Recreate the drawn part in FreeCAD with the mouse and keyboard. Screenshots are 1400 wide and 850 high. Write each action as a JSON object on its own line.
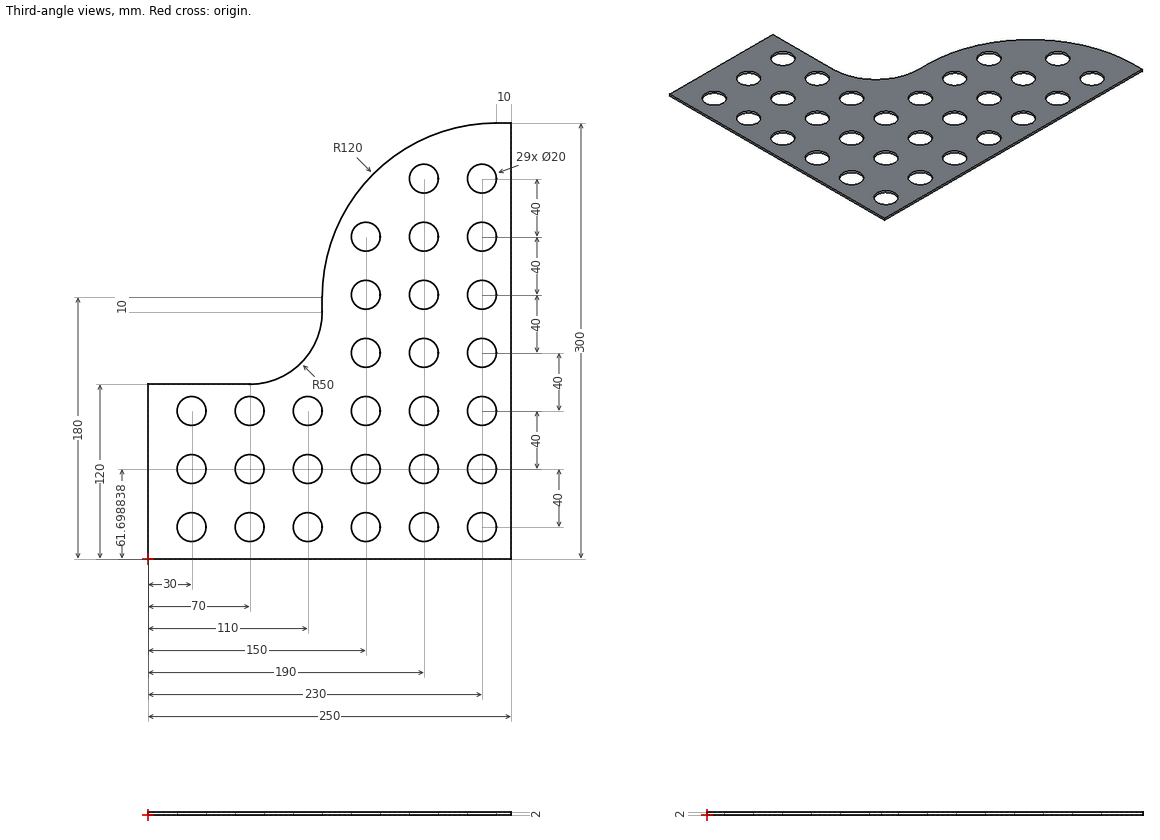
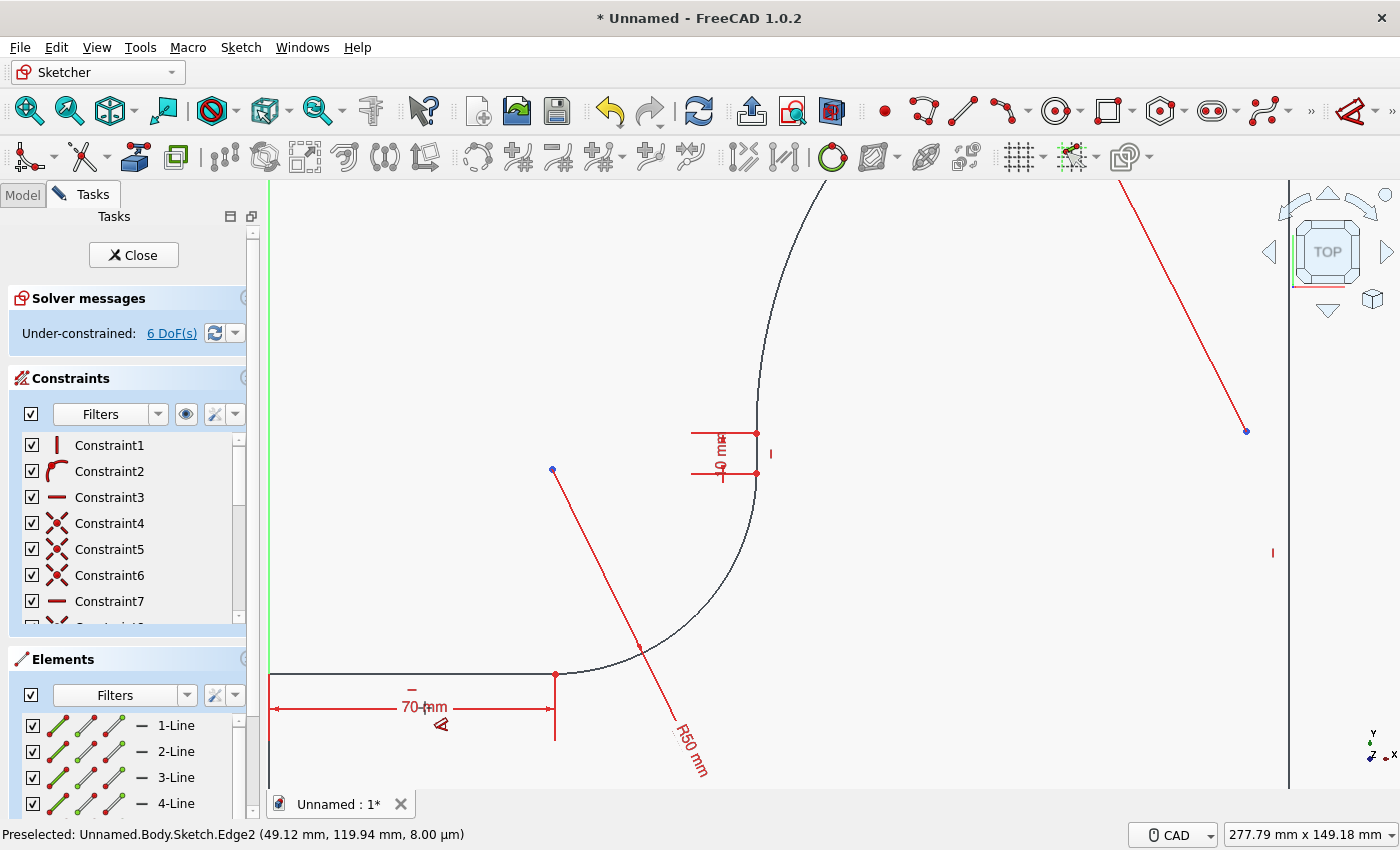
{"action": "scroll", "coordinate": [758, 456], "scroll_direction": "down", "scroll_amount": 6}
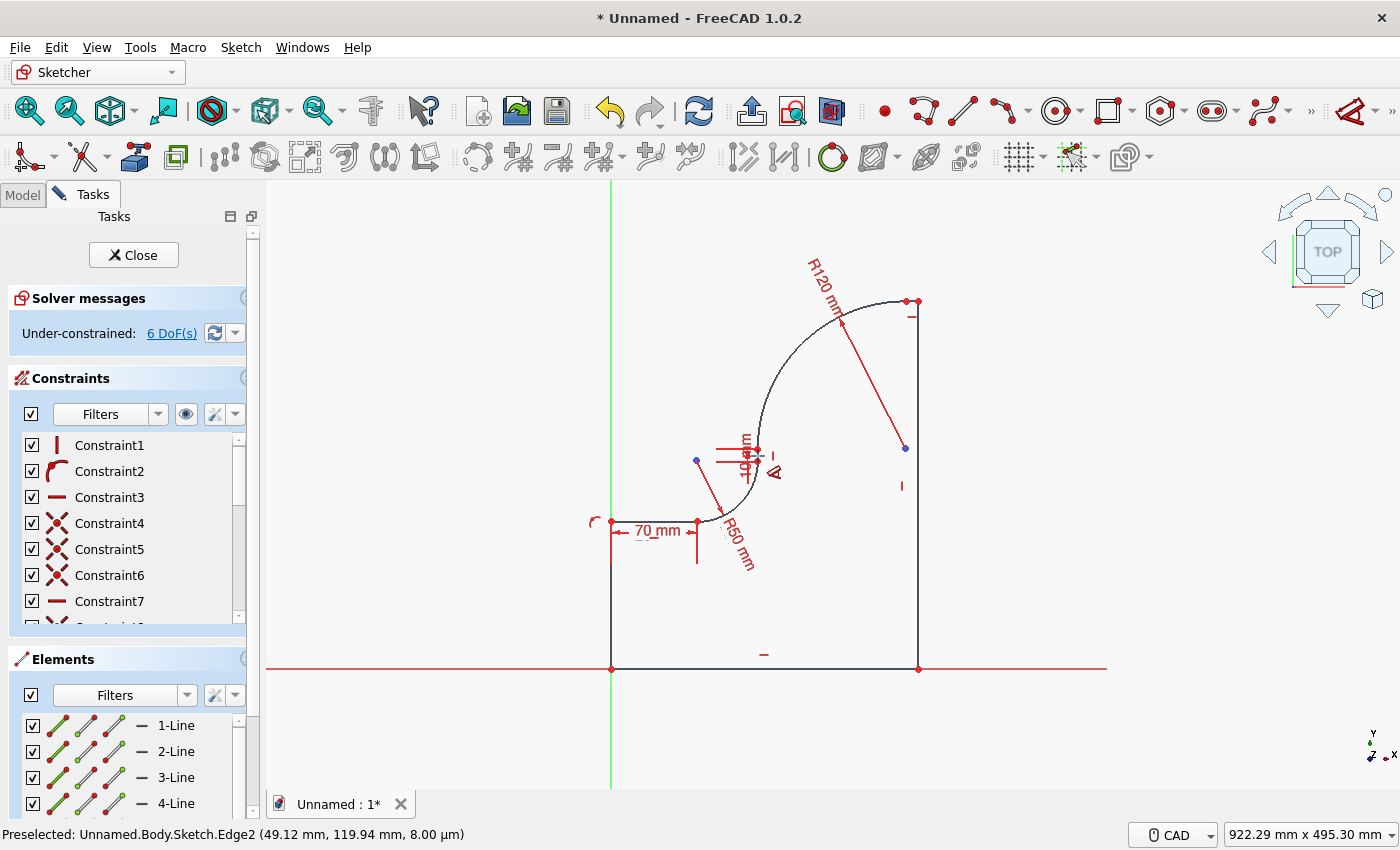
{"action": "scroll", "coordinate": [915, 301], "scroll_direction": "up", "scroll_amount": 7}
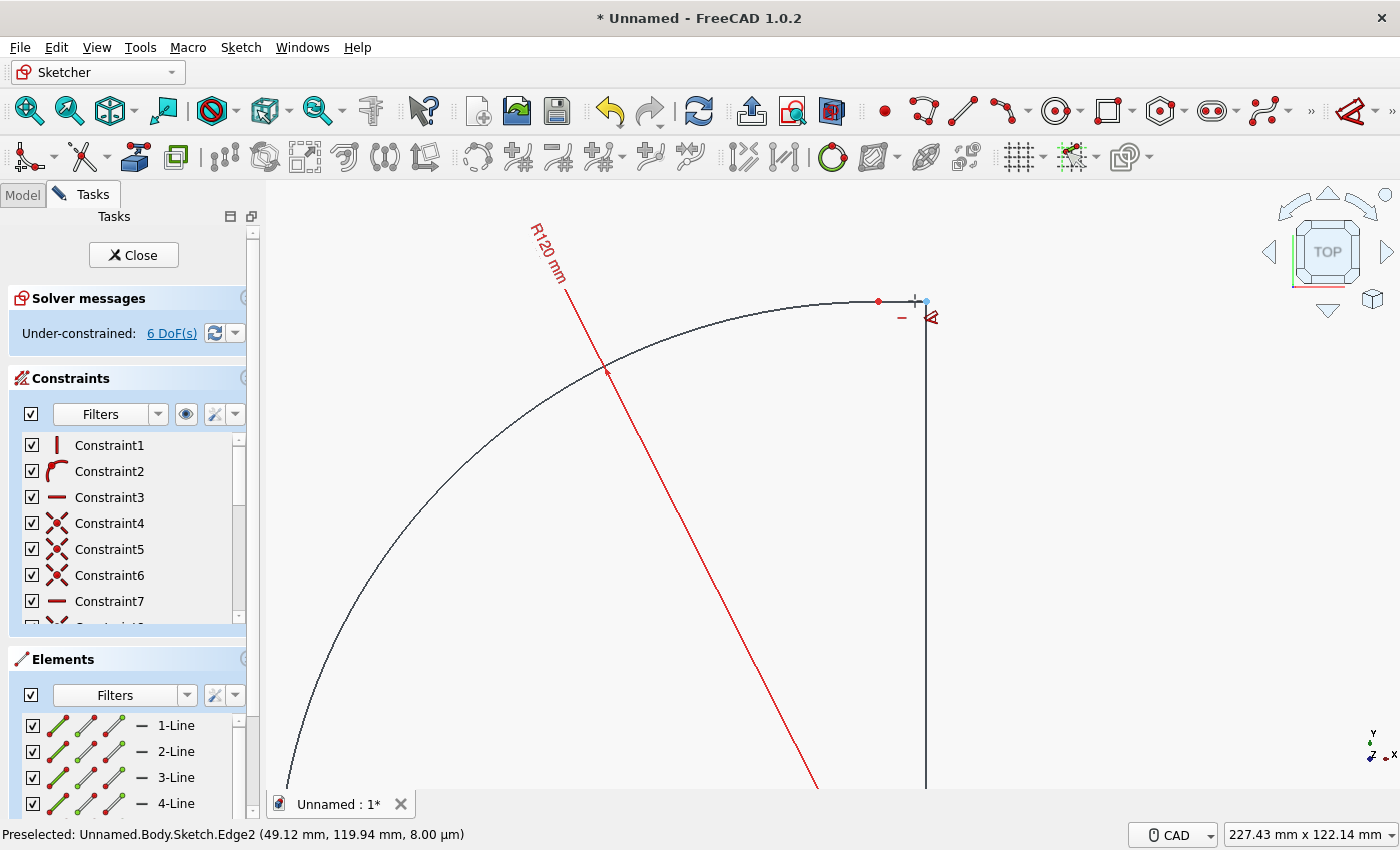
{"action": "left_click", "coordinate": [912, 302]}
{"action": "left_click", "coordinate": [902, 268]}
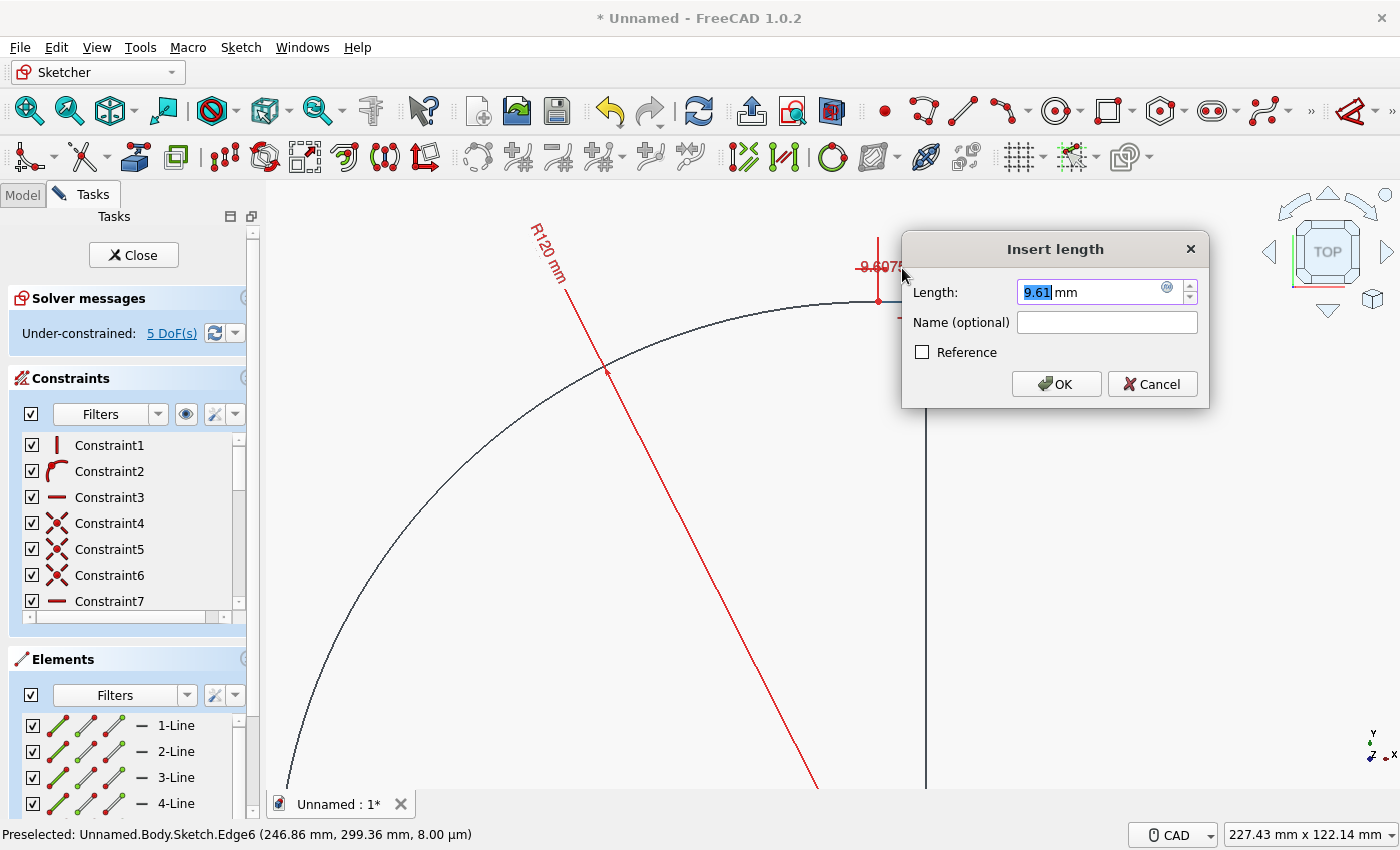
{"action": "type", "text": "10"}
{"action": "key", "text": "Return"}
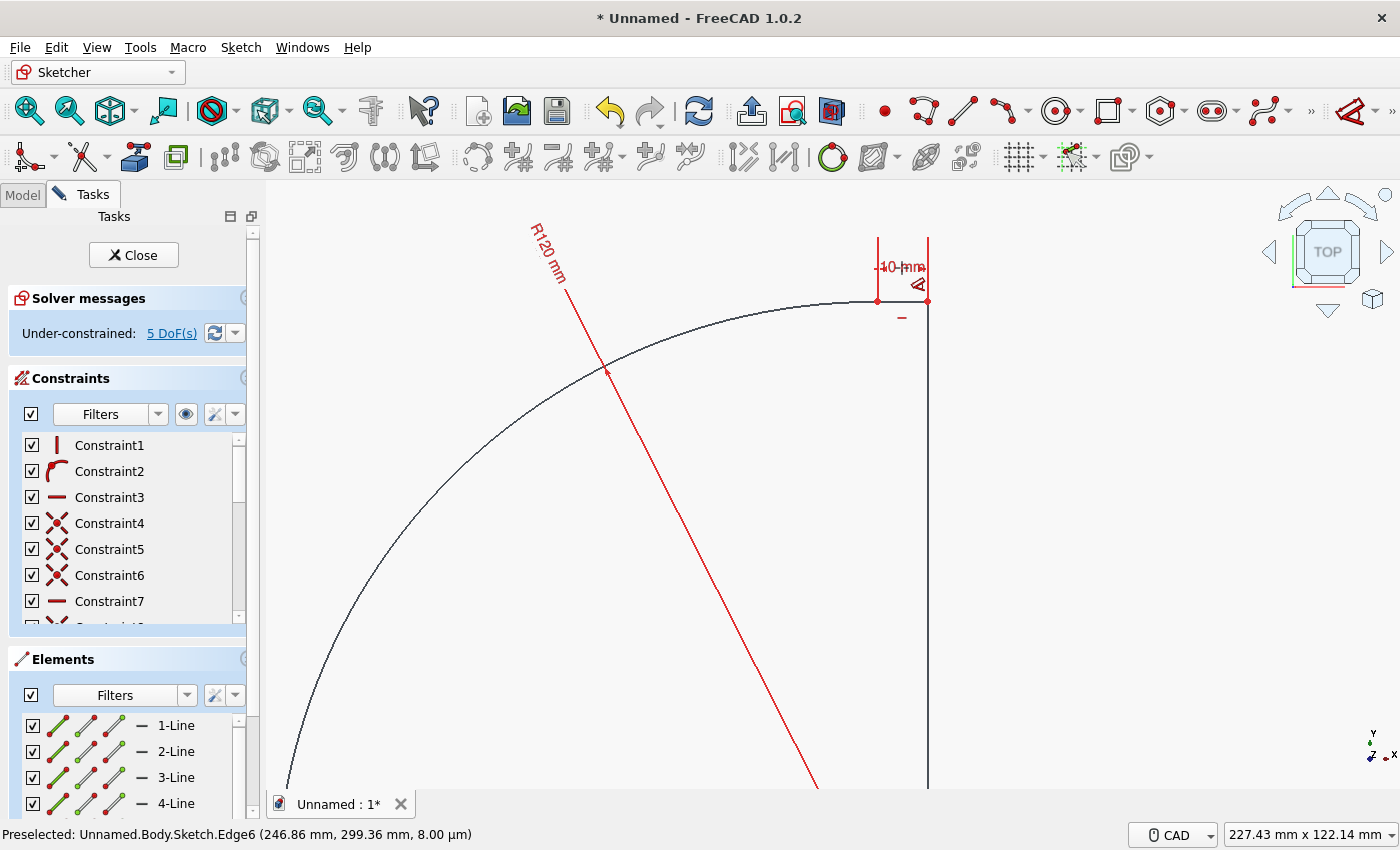
{"action": "scroll", "coordinate": [915, 301], "scroll_direction": "down", "scroll_amount": 7}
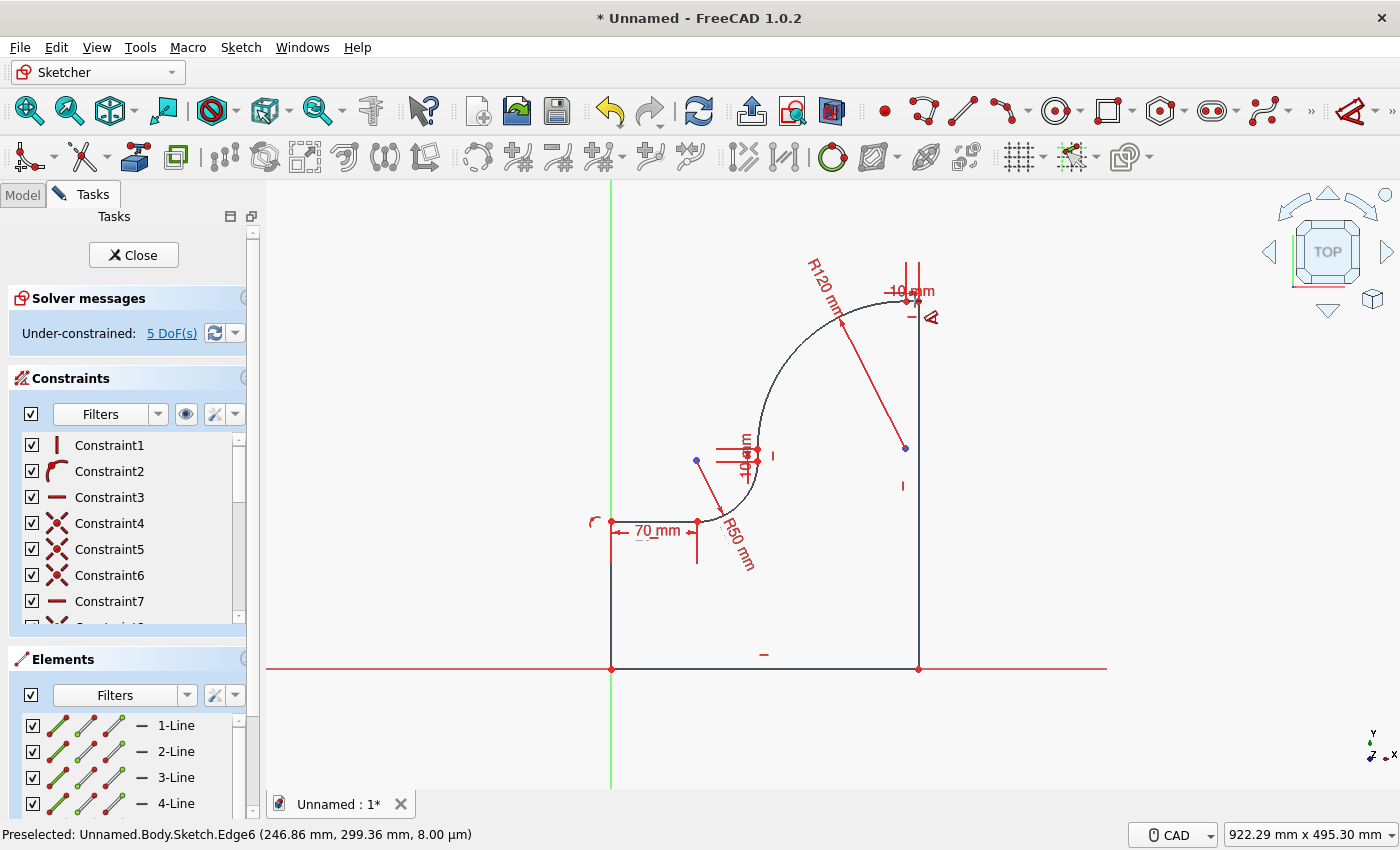
{"action": "left_click", "coordinate": [611, 566]}
{"action": "left_click", "coordinate": [577, 596]}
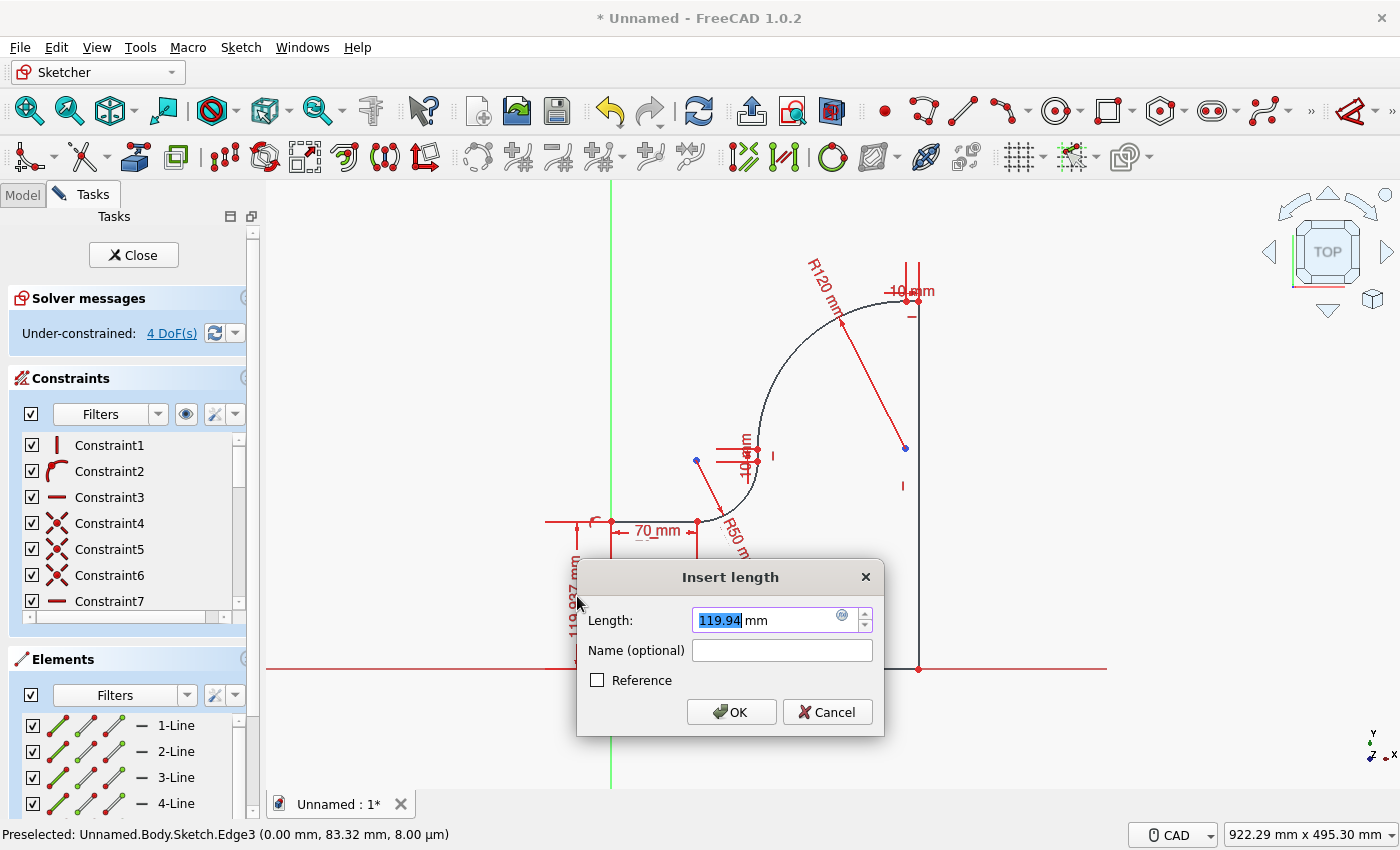
{"action": "type", "text": "120"}
{"action": "key", "text": "Return"}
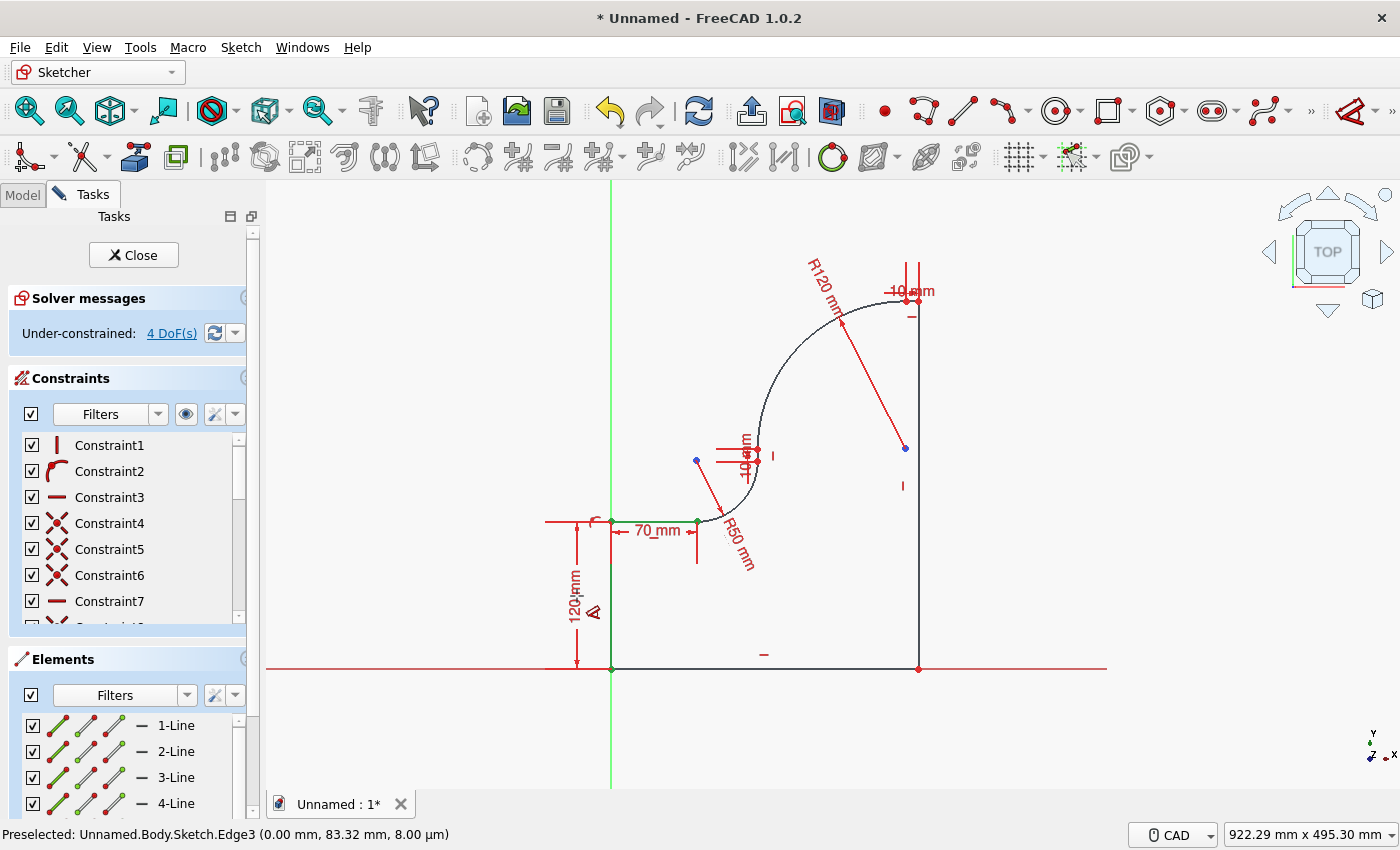
{"action": "left_click", "coordinate": [703, 669]}
{"action": "left_click", "coordinate": [765, 703]}